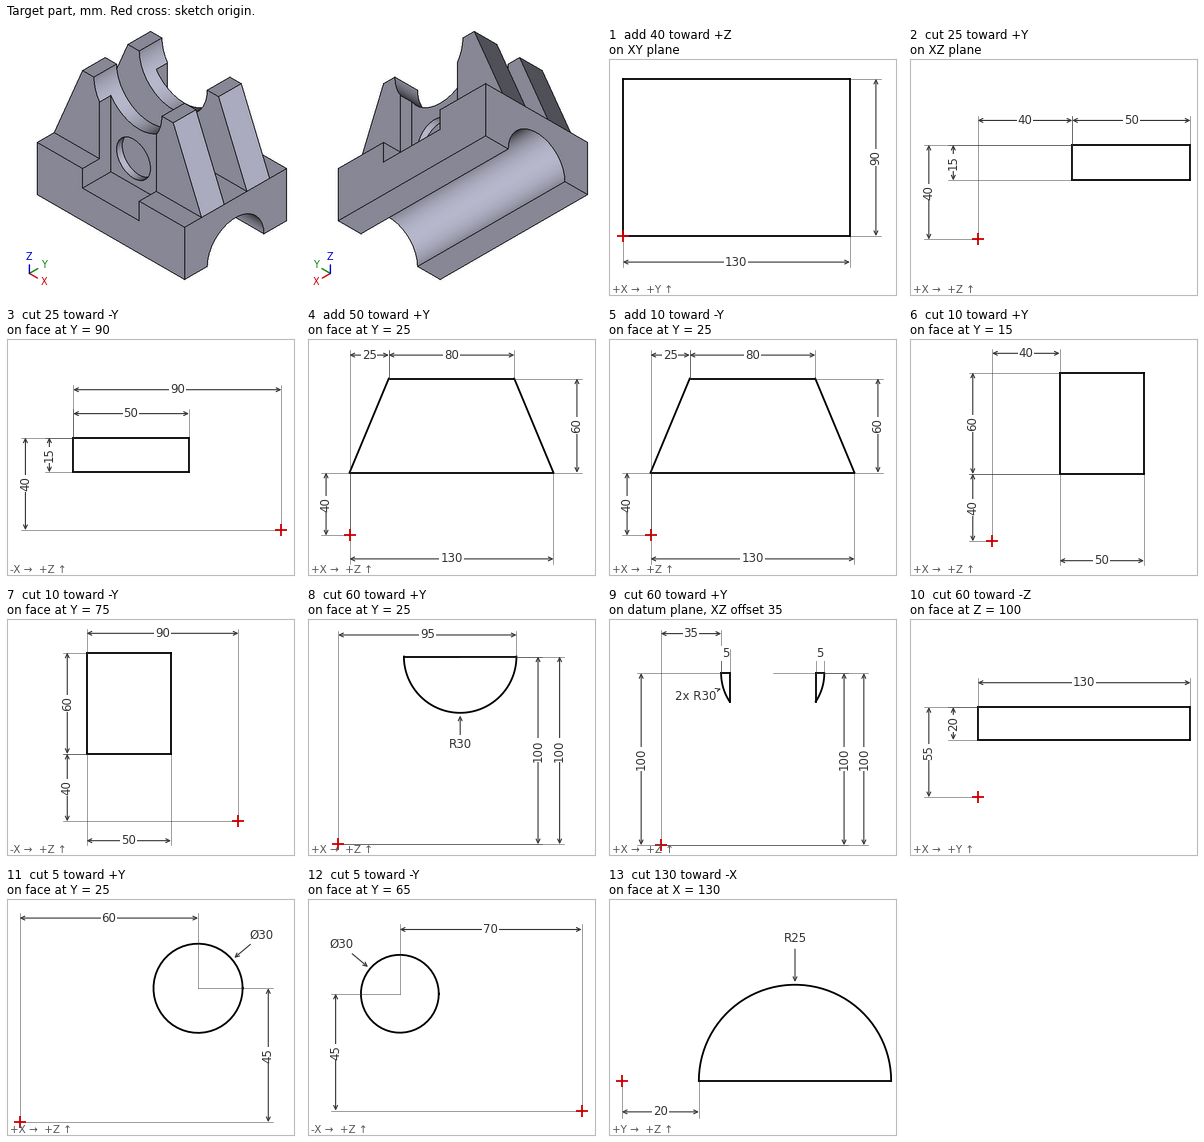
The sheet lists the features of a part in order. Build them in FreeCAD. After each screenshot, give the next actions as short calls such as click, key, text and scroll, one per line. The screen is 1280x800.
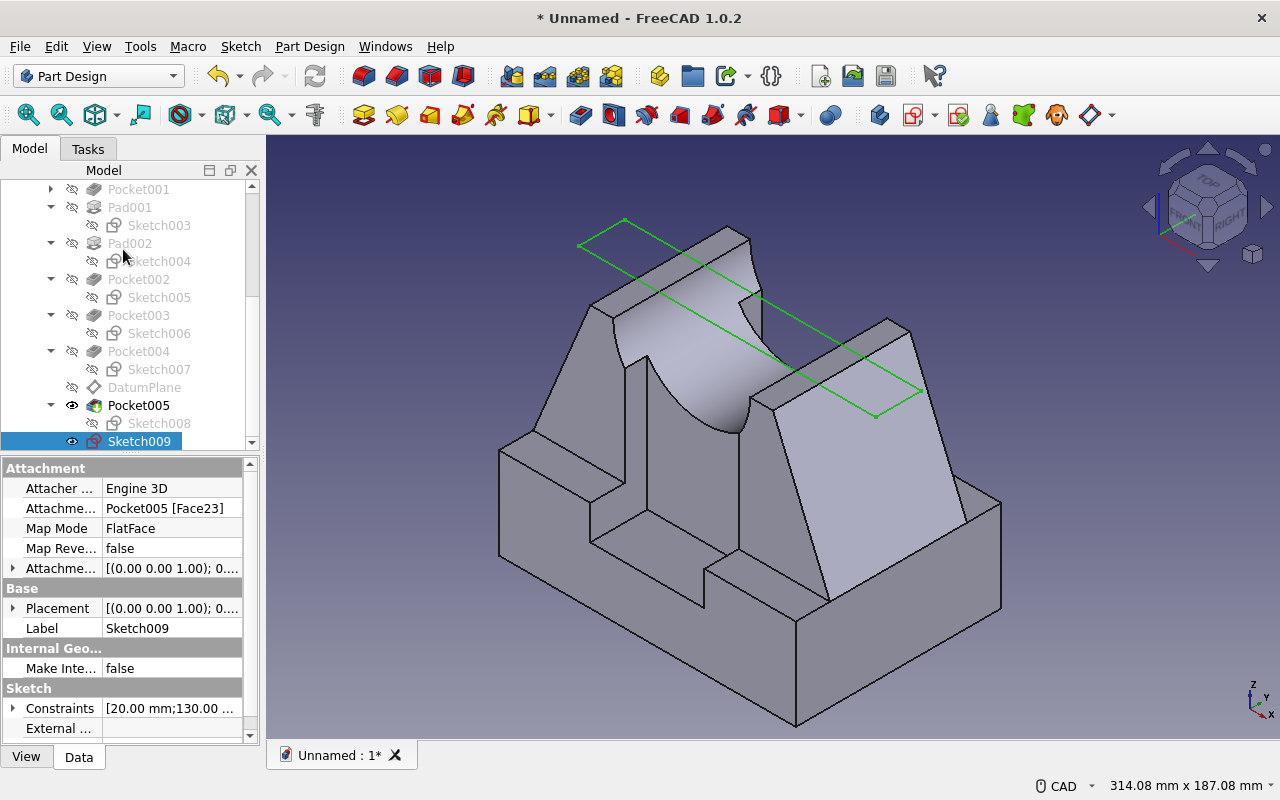
click(581, 116)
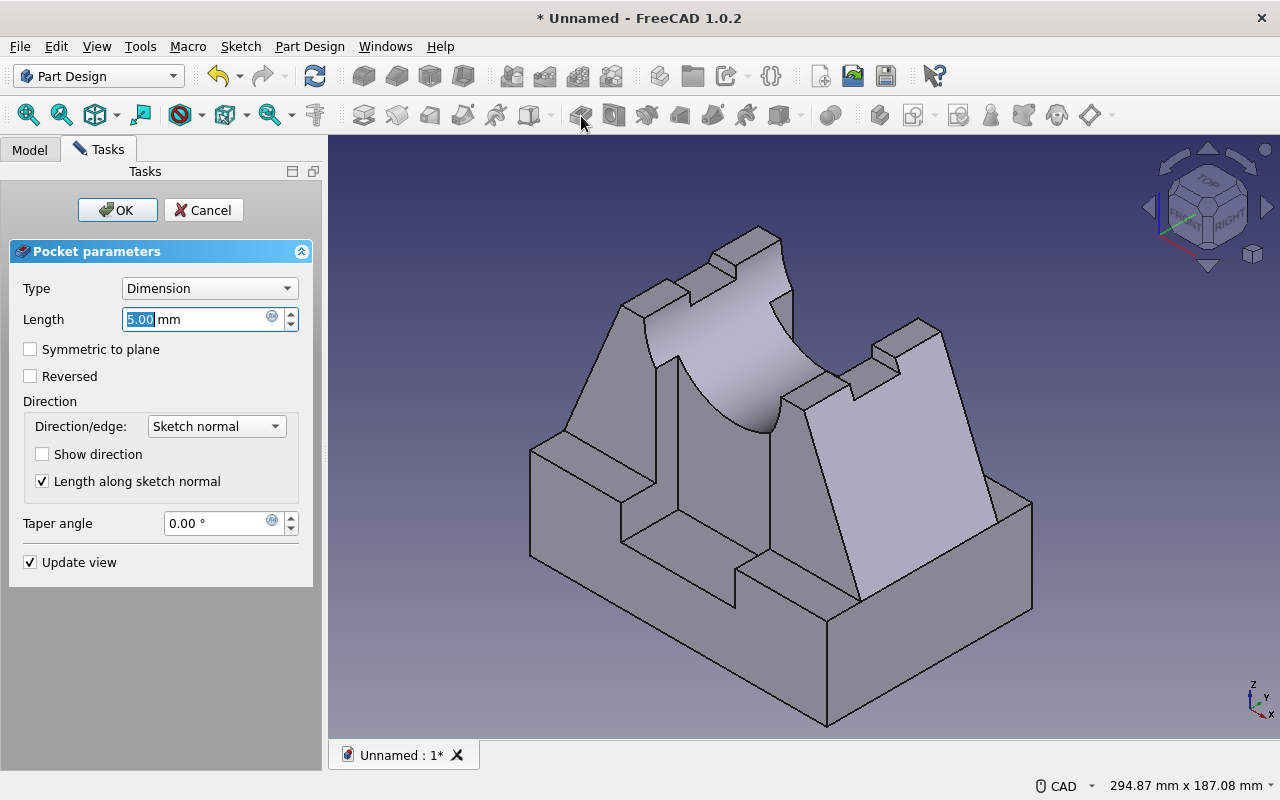
text(60)
key(Tab)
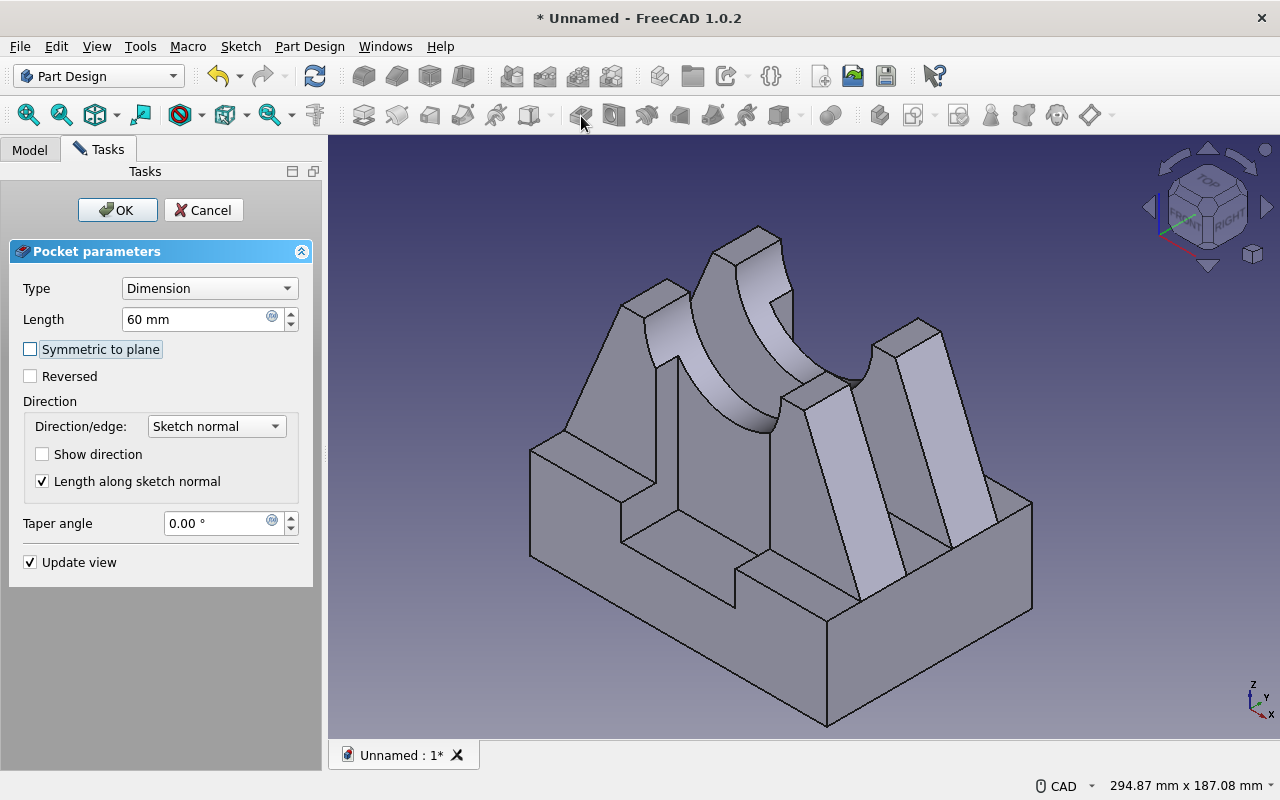
click(118, 210)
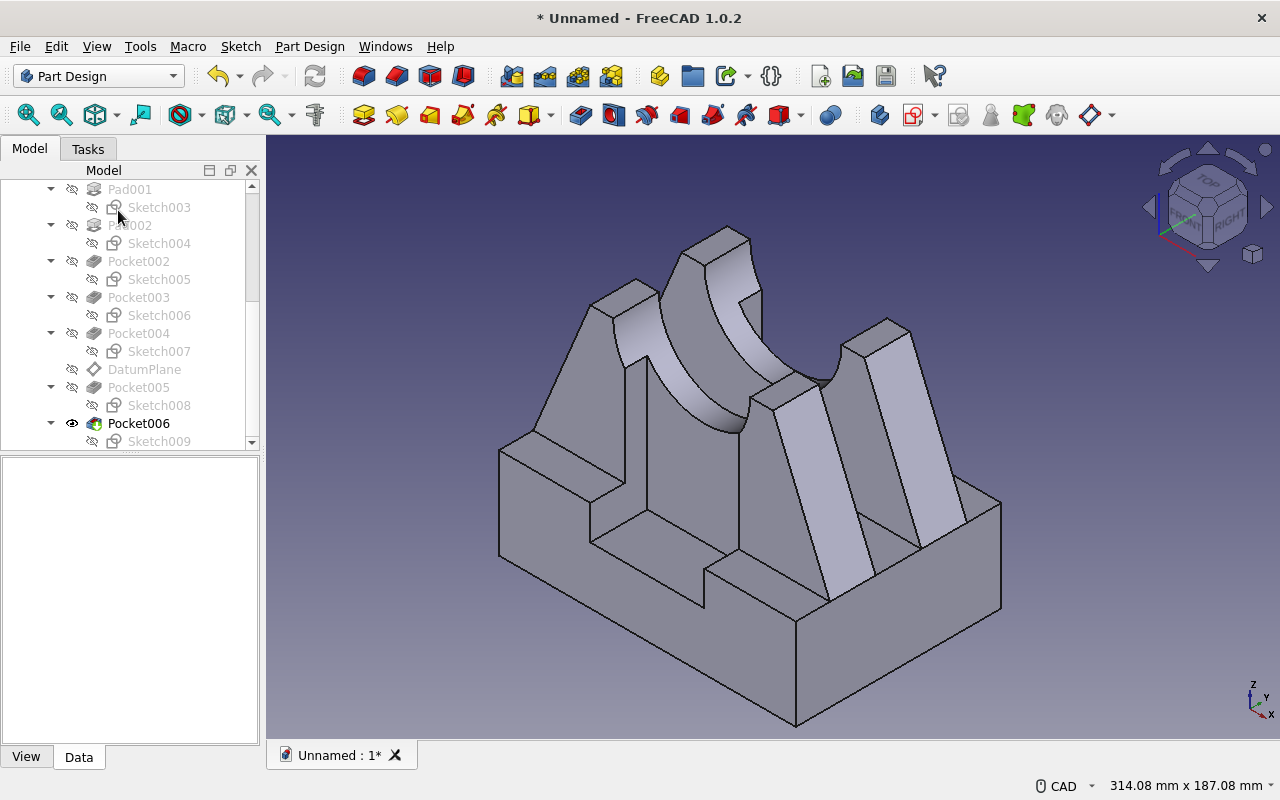
click(704, 486)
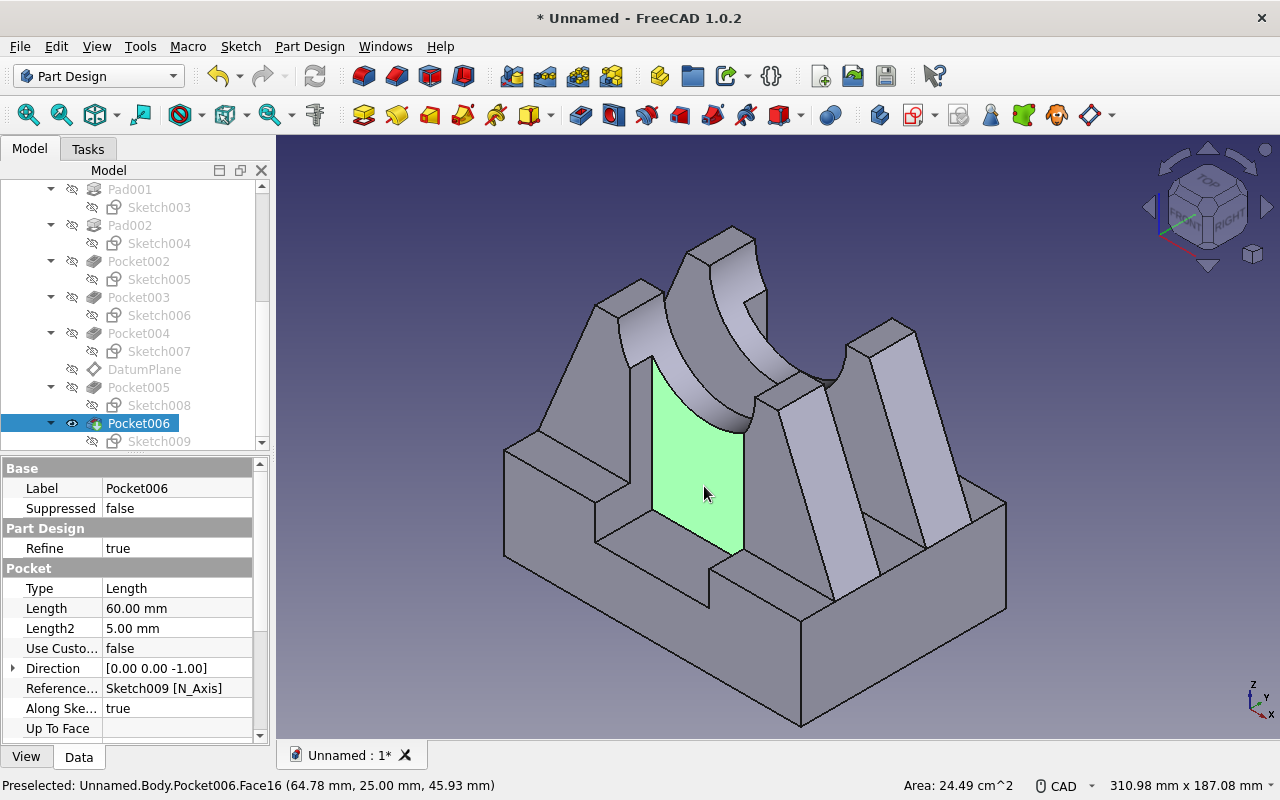
click(912, 116)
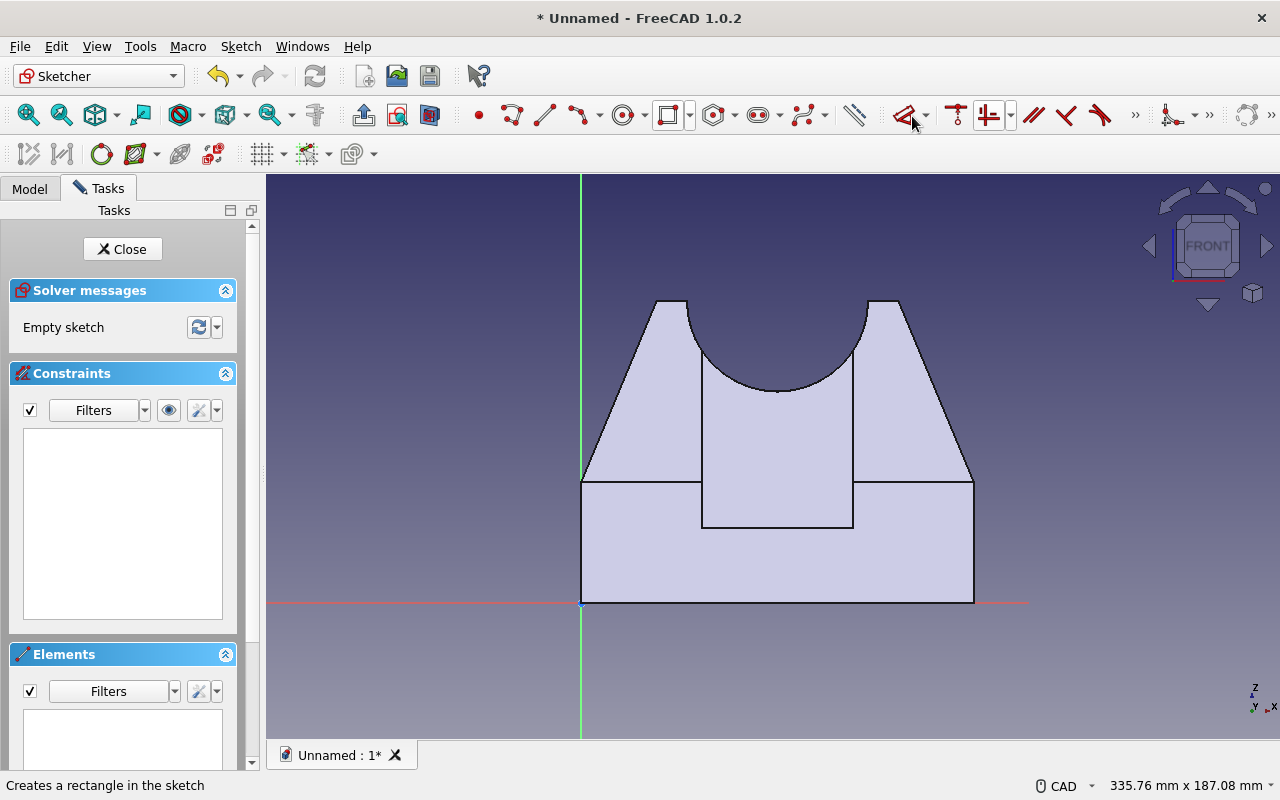
scroll(781, 471, up, 7)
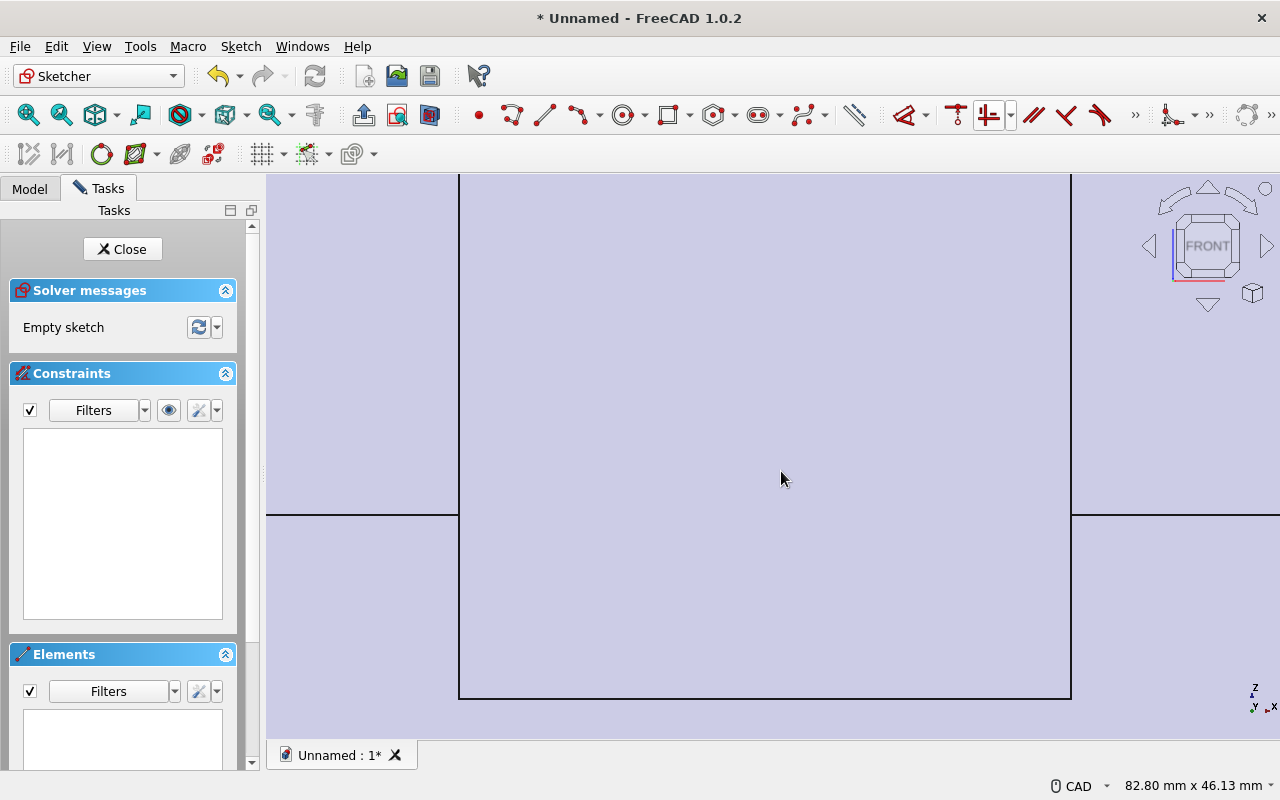
key(g)
key(c)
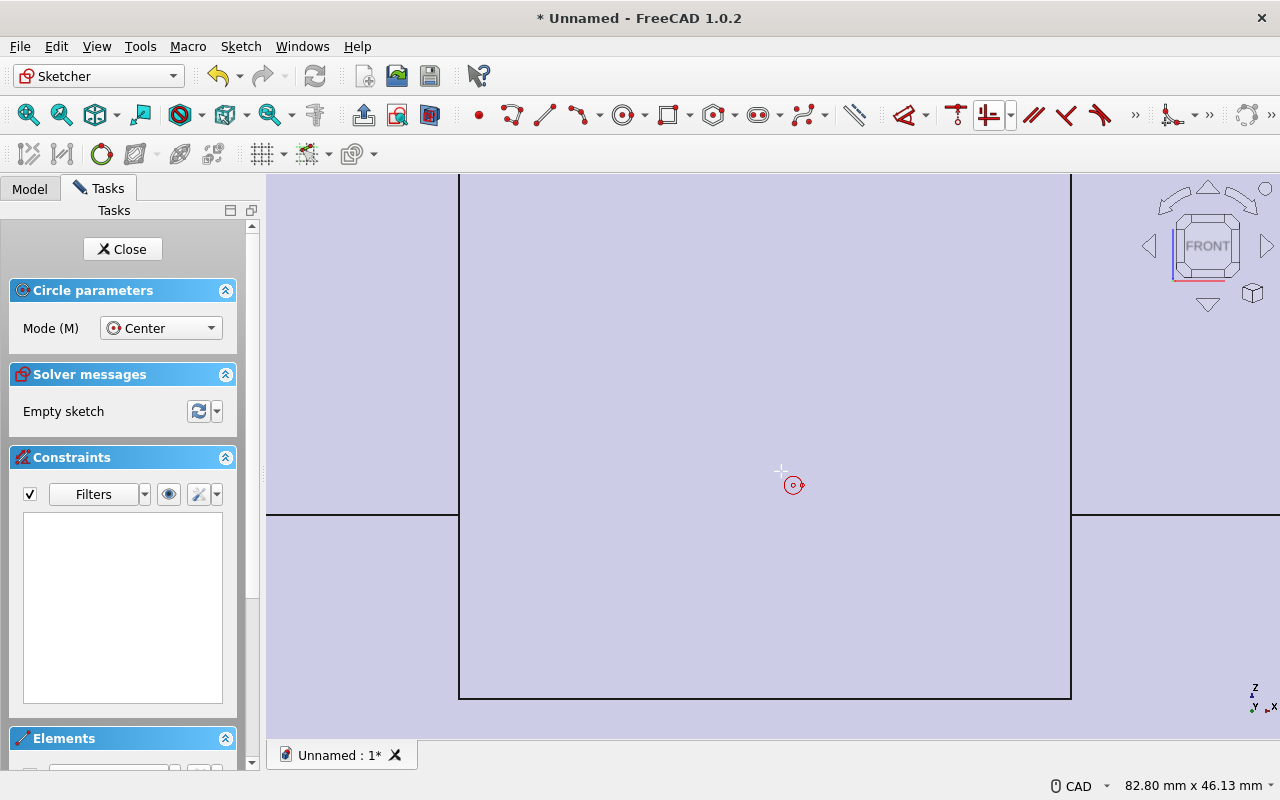
click(704, 454)
click(834, 324)
key(Escape)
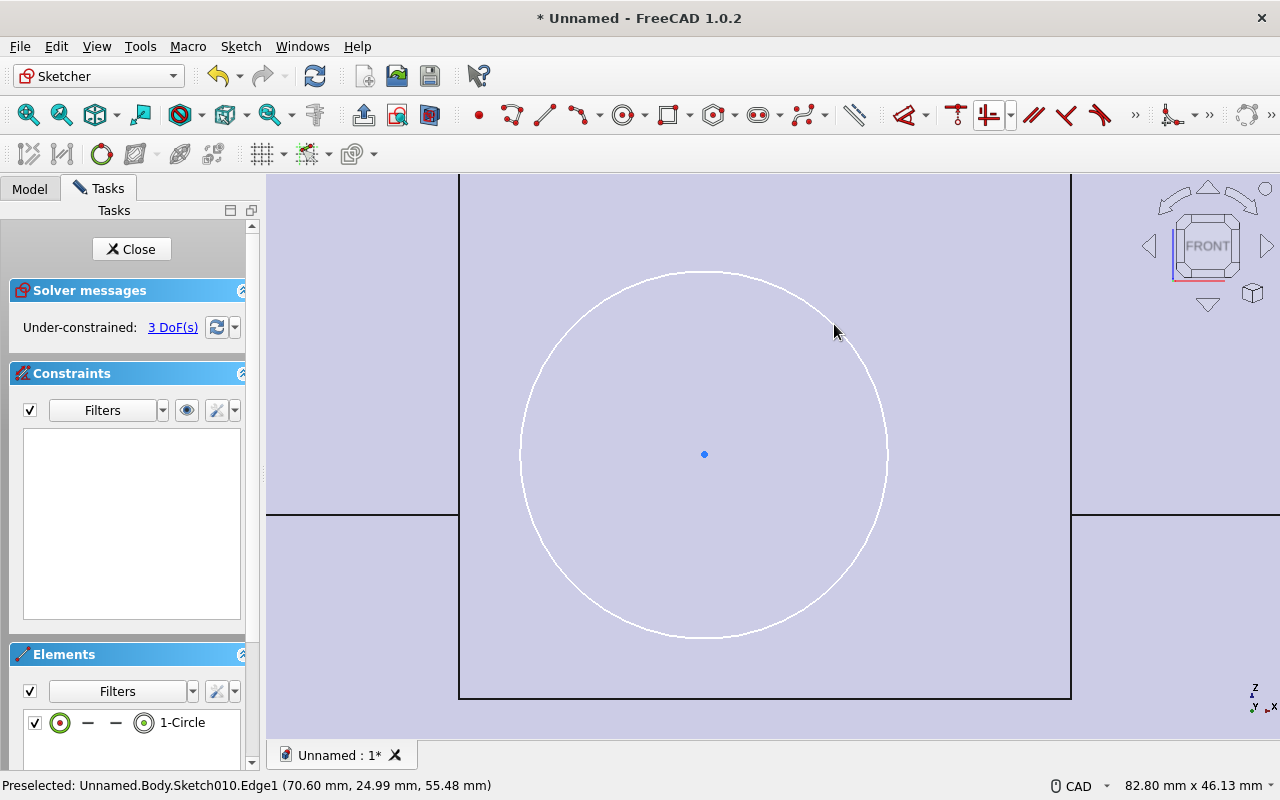
key(d)